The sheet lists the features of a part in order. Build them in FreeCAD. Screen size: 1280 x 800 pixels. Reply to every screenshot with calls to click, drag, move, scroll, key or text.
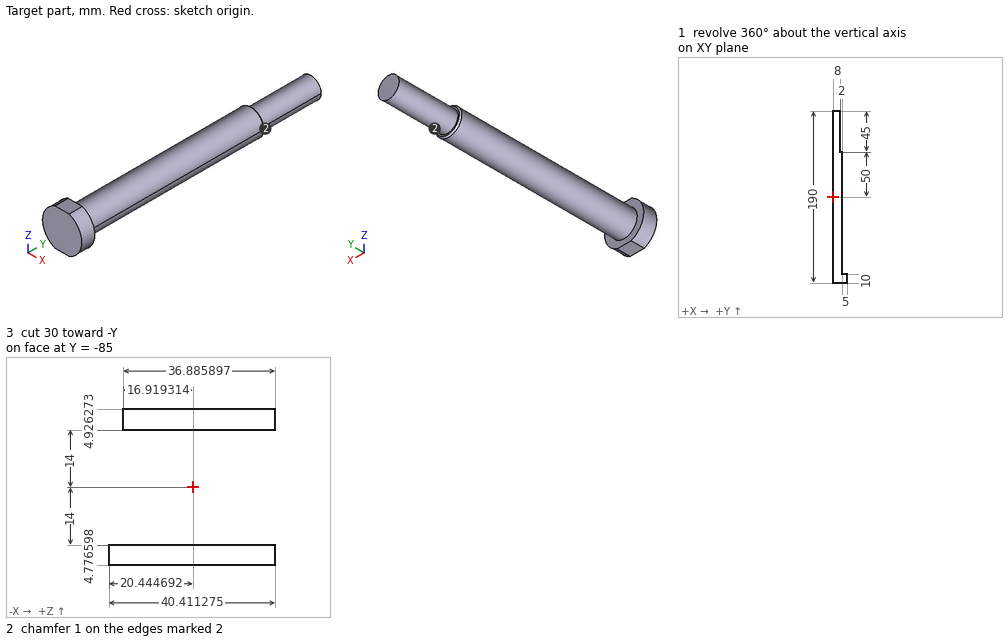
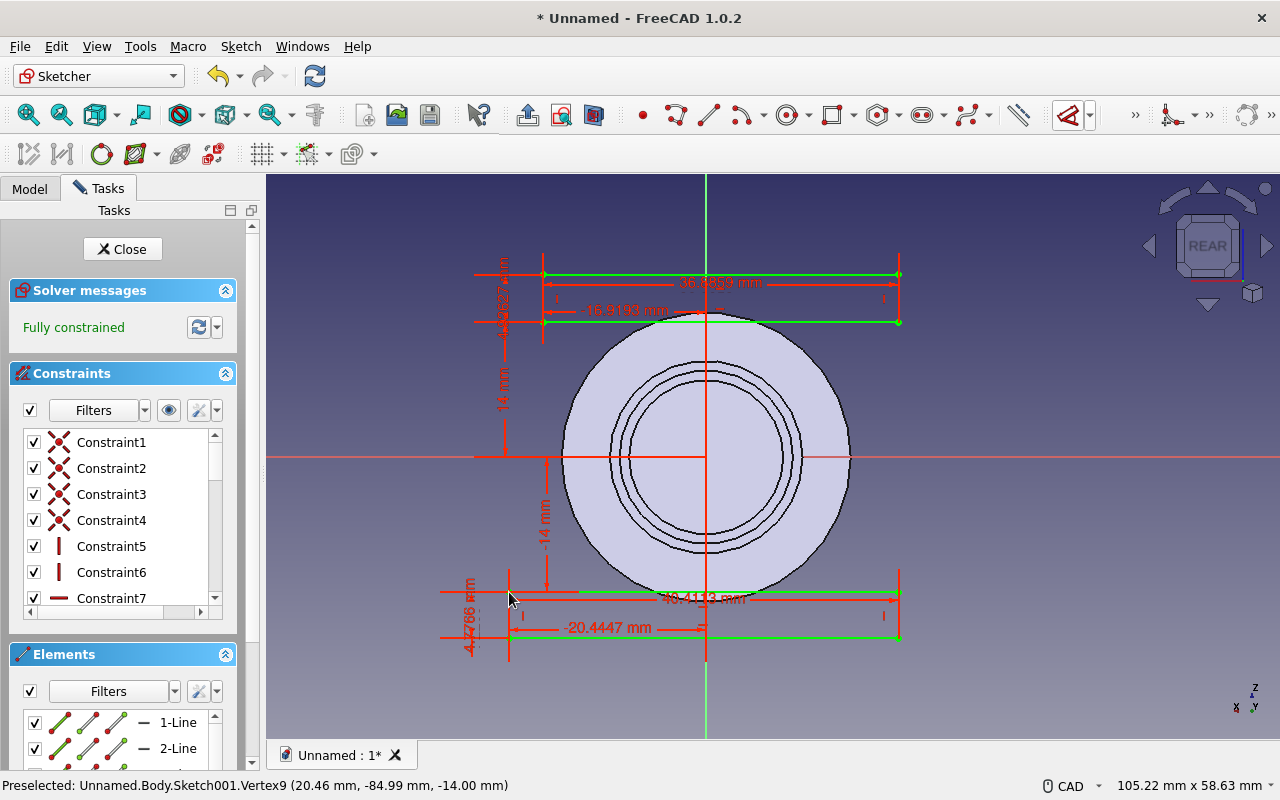
click(123, 249)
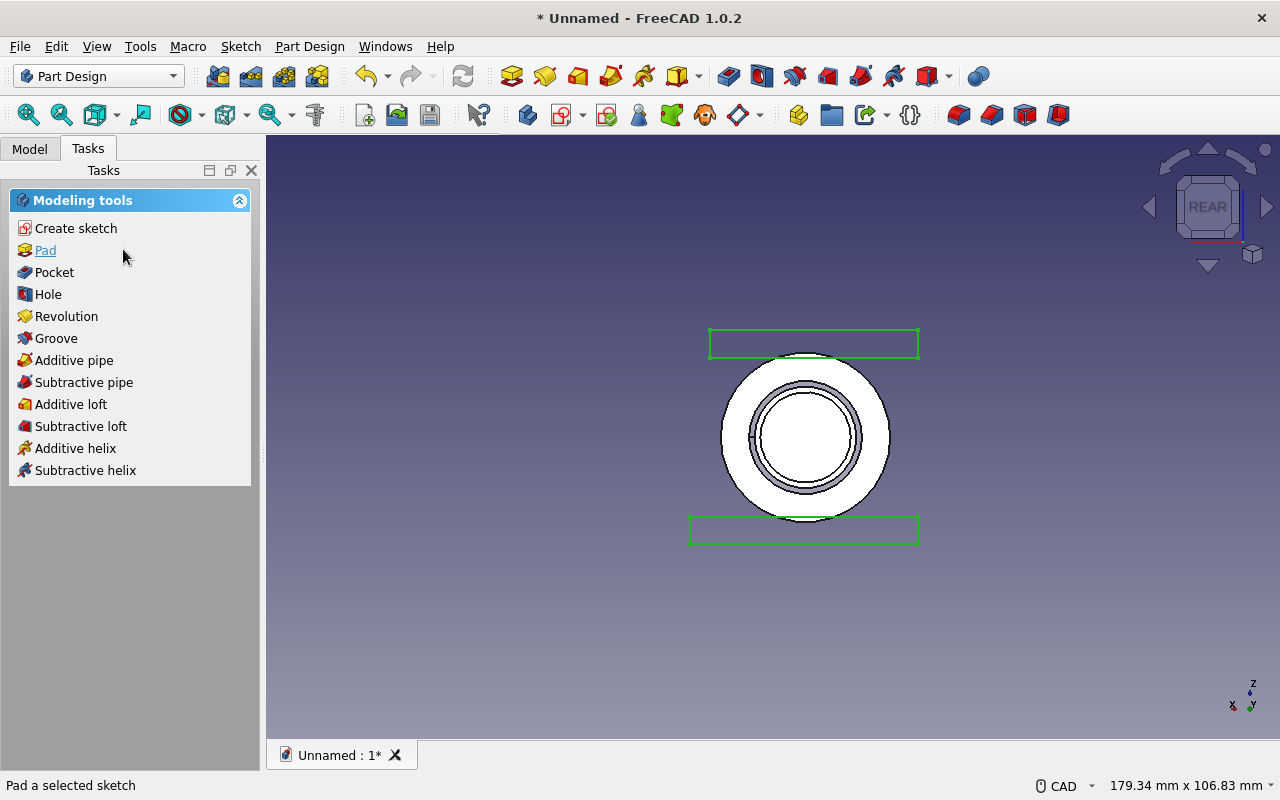
click(729, 76)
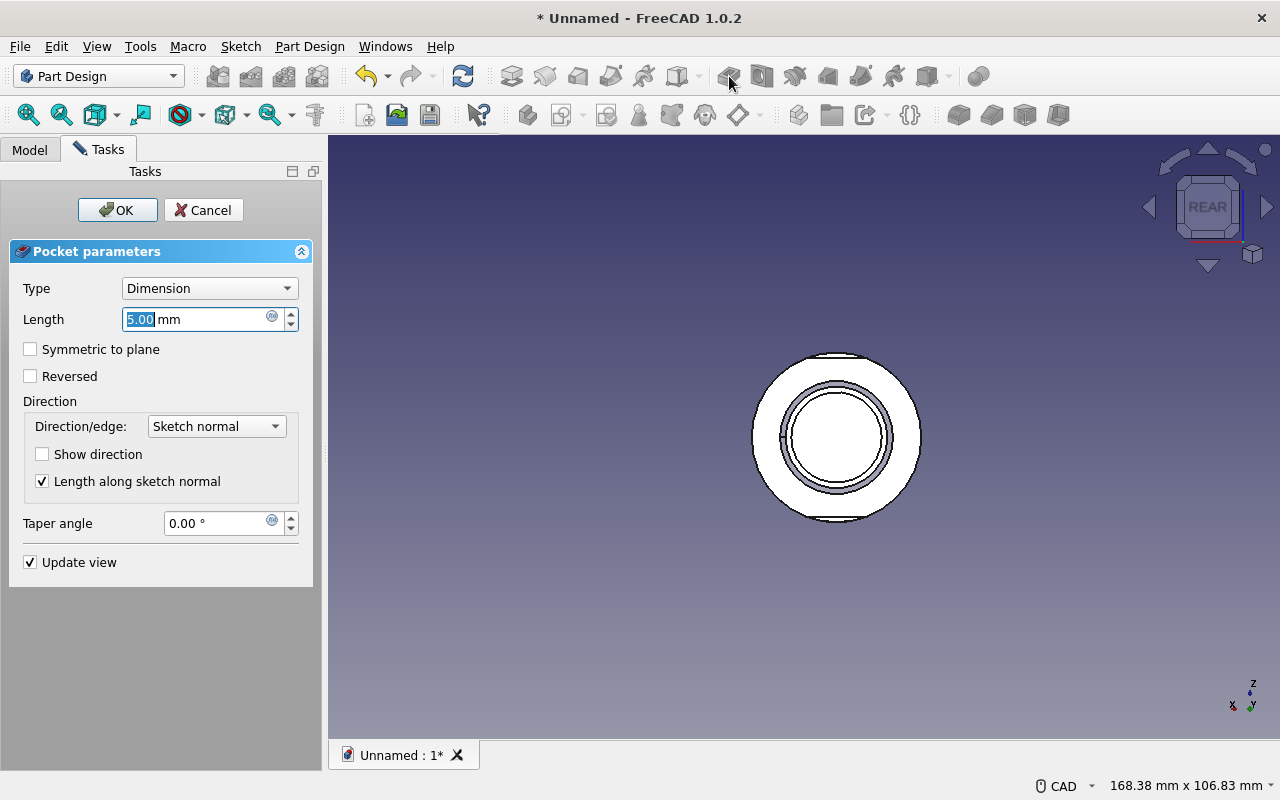
text(30)
key(Tab)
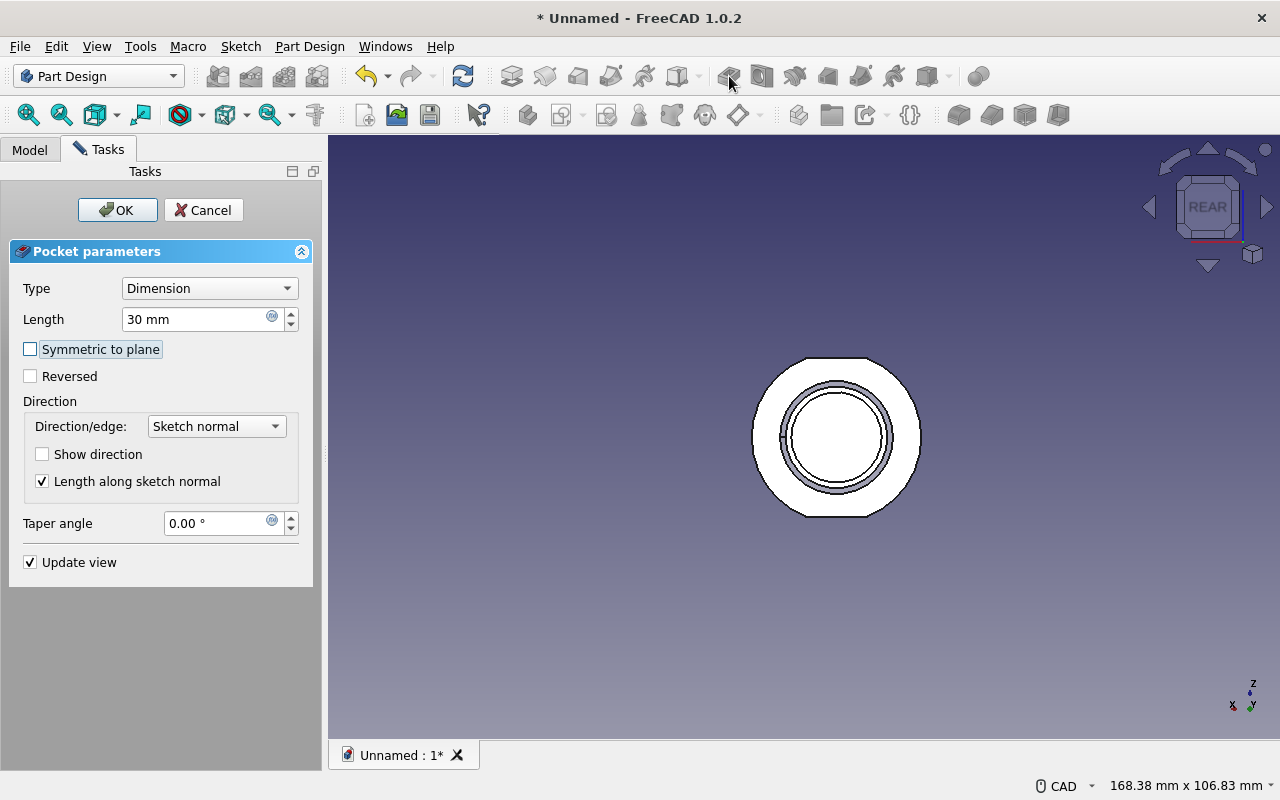
click(118, 210)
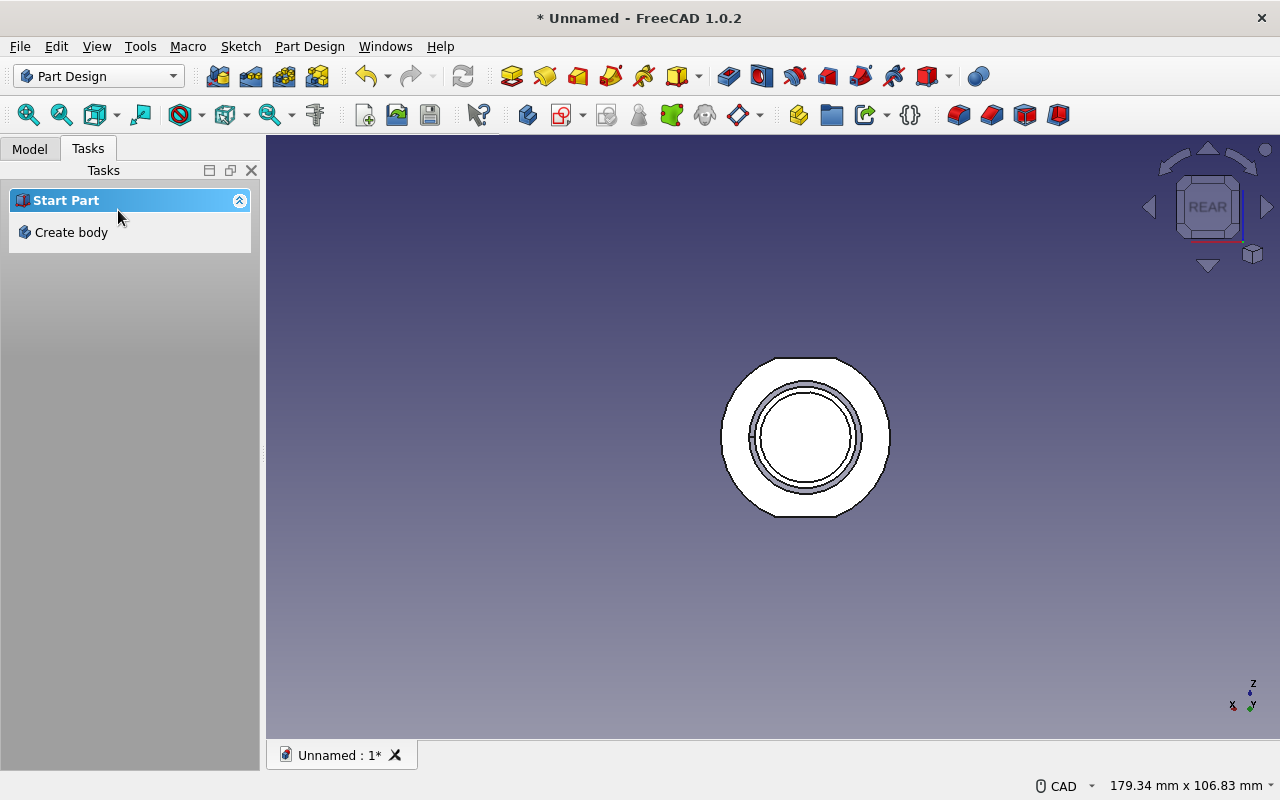
key(0)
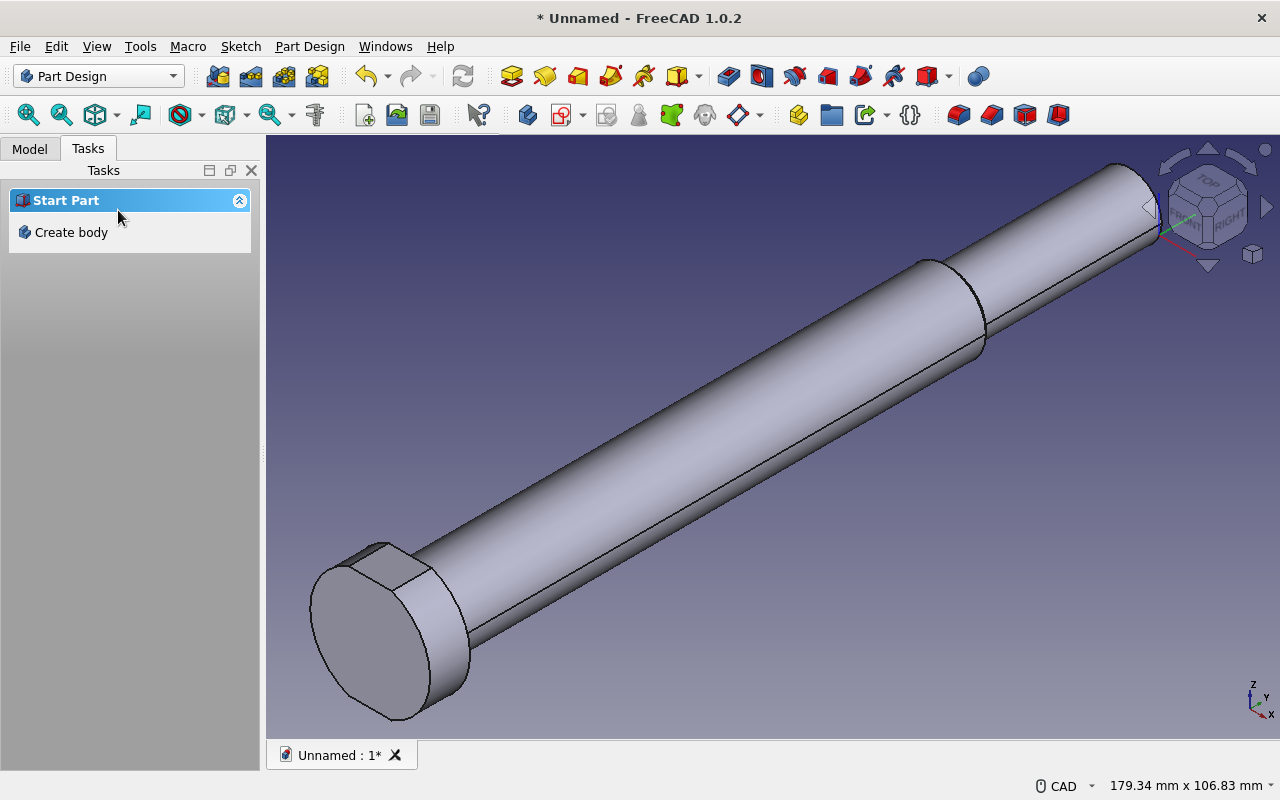
click(29, 116)